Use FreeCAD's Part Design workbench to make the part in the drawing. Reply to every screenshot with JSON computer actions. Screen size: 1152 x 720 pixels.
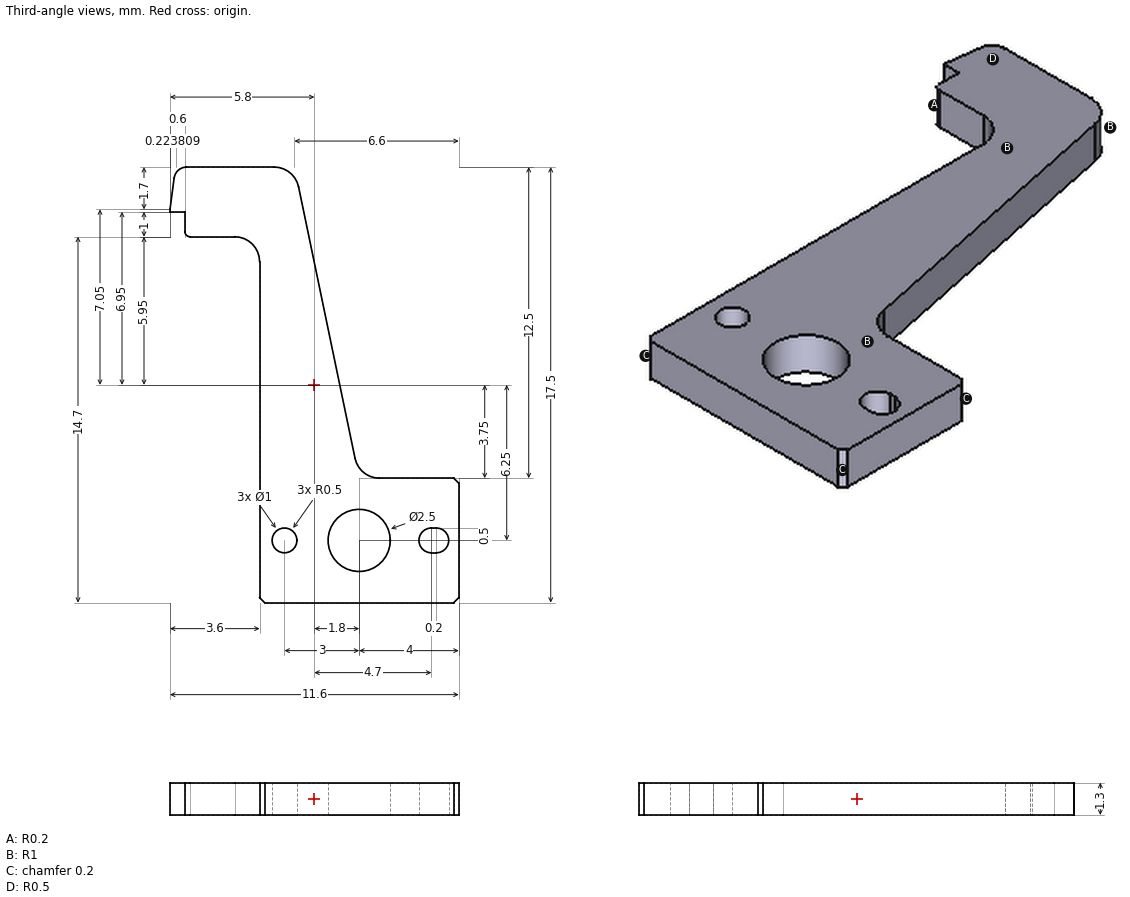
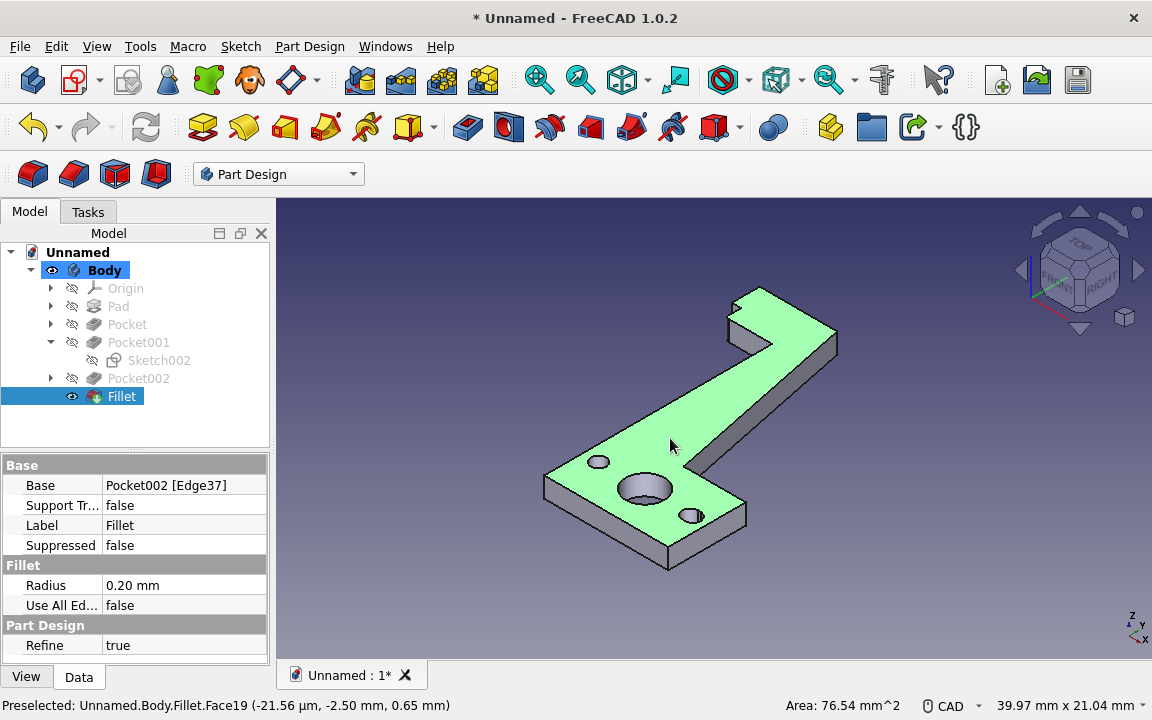
{"action": "left_click", "coordinate": [74, 80]}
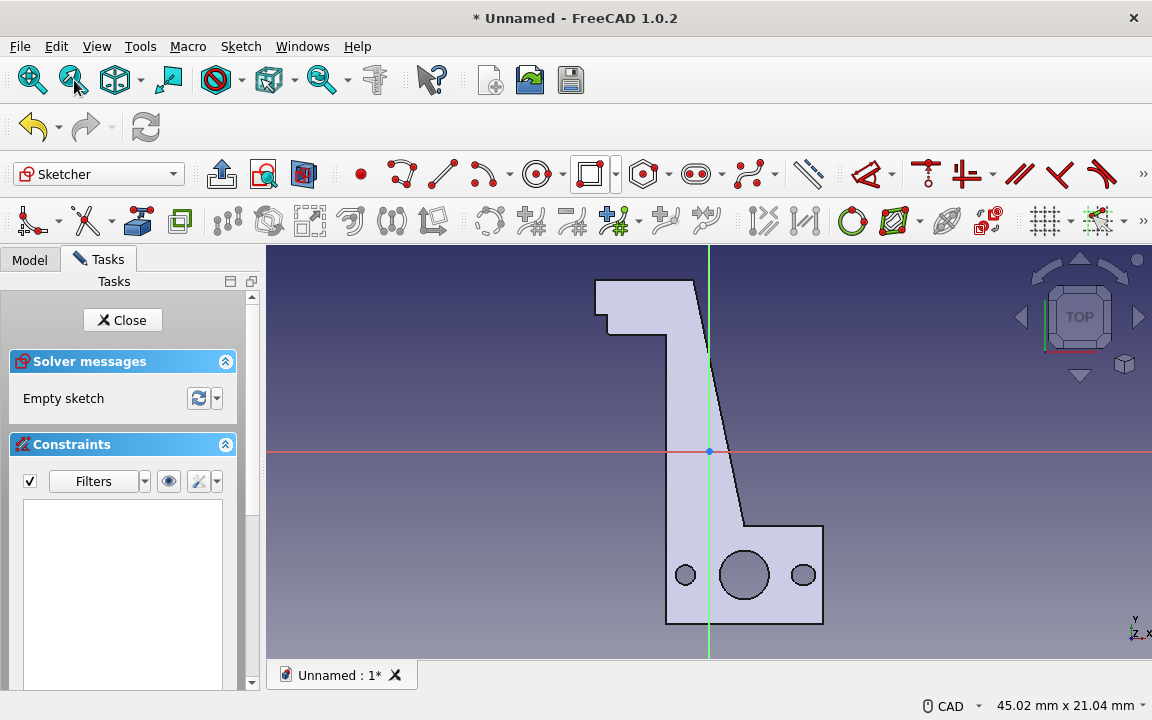
{"action": "scroll", "coordinate": [590, 273], "scroll_direction": "up", "scroll_amount": 10}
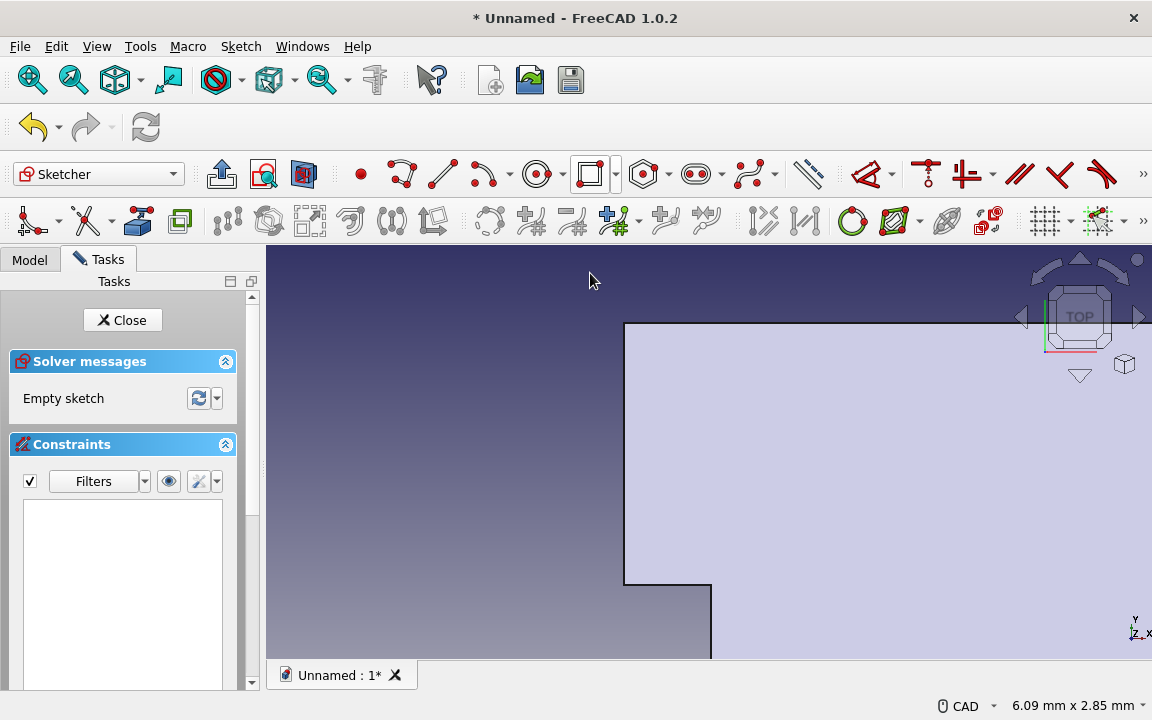
{"action": "key", "text": "g m"}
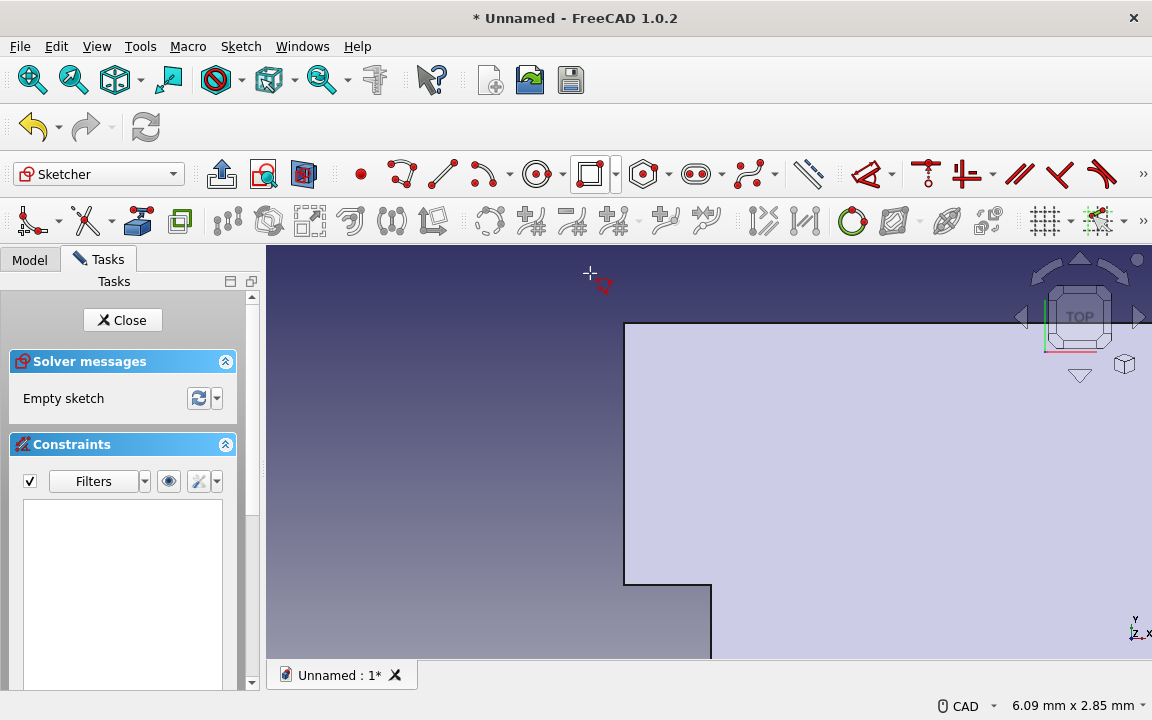
{"action": "left_click", "coordinate": [624, 570]}
{"action": "left_click", "coordinate": [656, 323]}
{"action": "left_click", "coordinate": [624, 323]}
{"action": "left_click", "coordinate": [624, 571]}
{"action": "key", "text": "Escape"}
{"action": "key", "text": "Escape"}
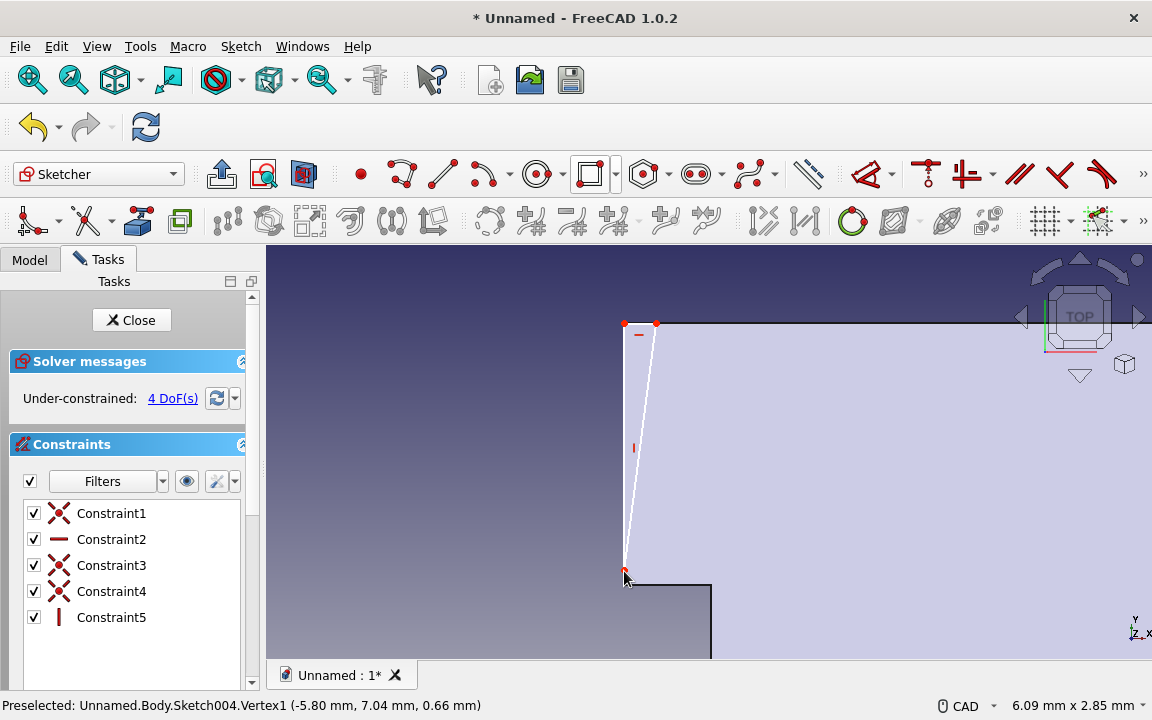
{"action": "key", "text": "d"}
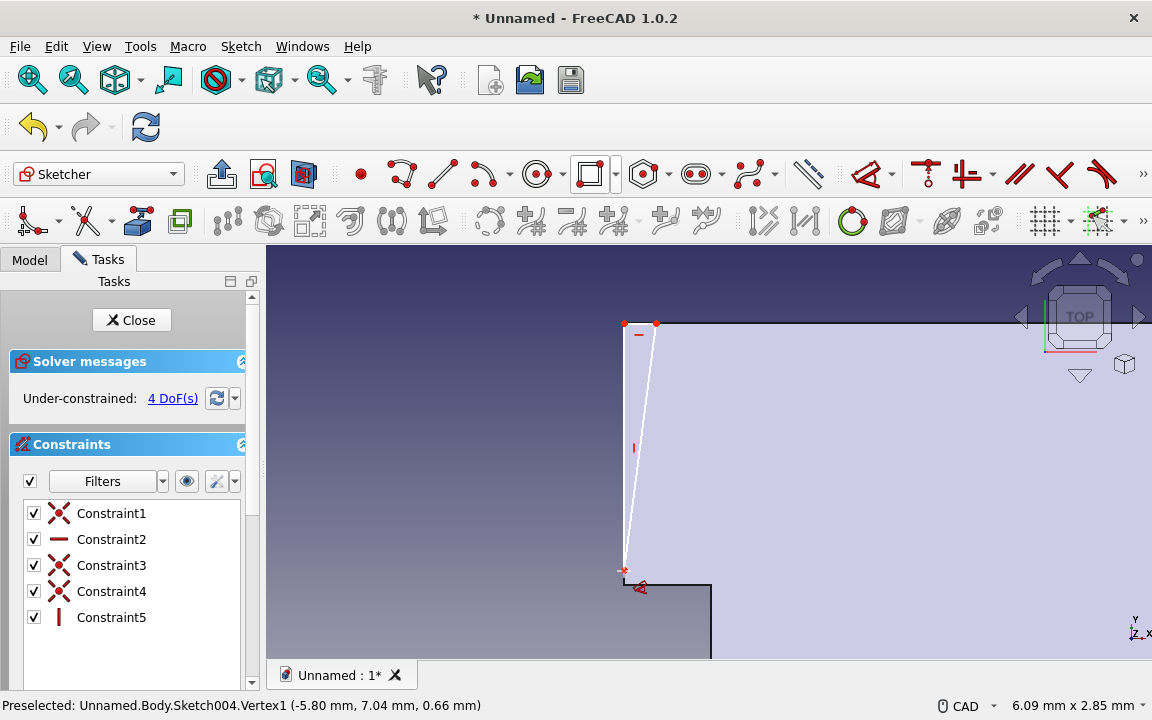
{"action": "left_click", "coordinate": [624, 398]}
{"action": "left_click", "coordinate": [590, 447]}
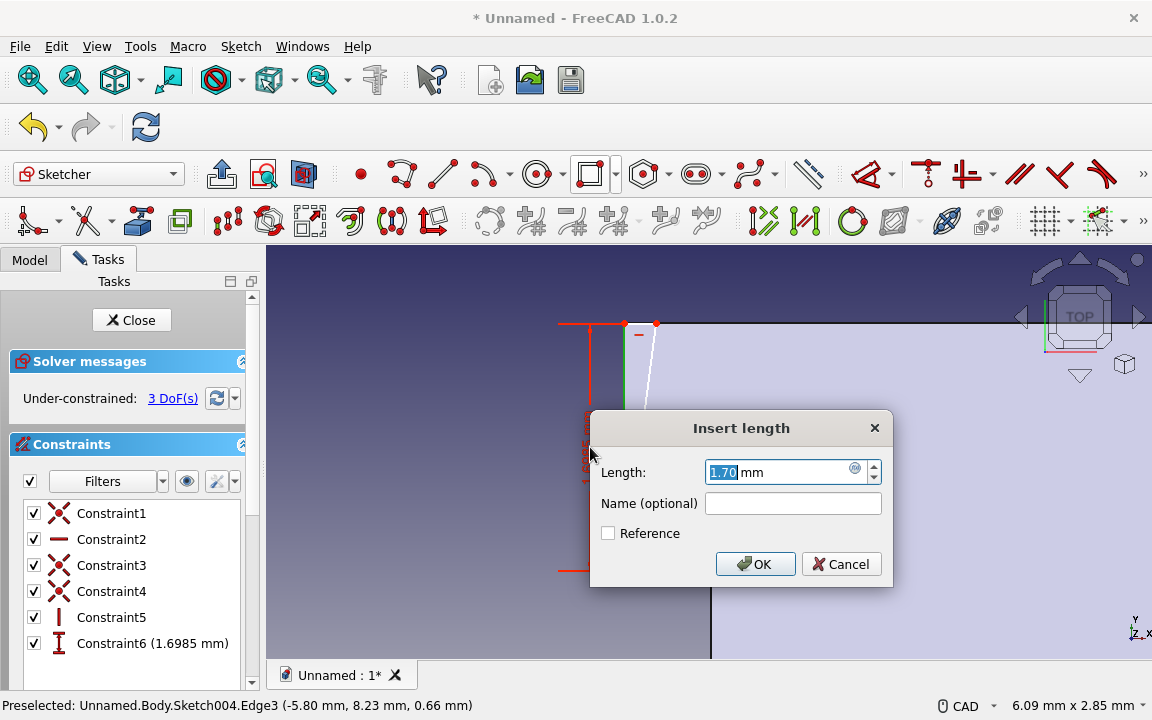
{"action": "type", "text": "1.7"}
{"action": "key", "text": "Return"}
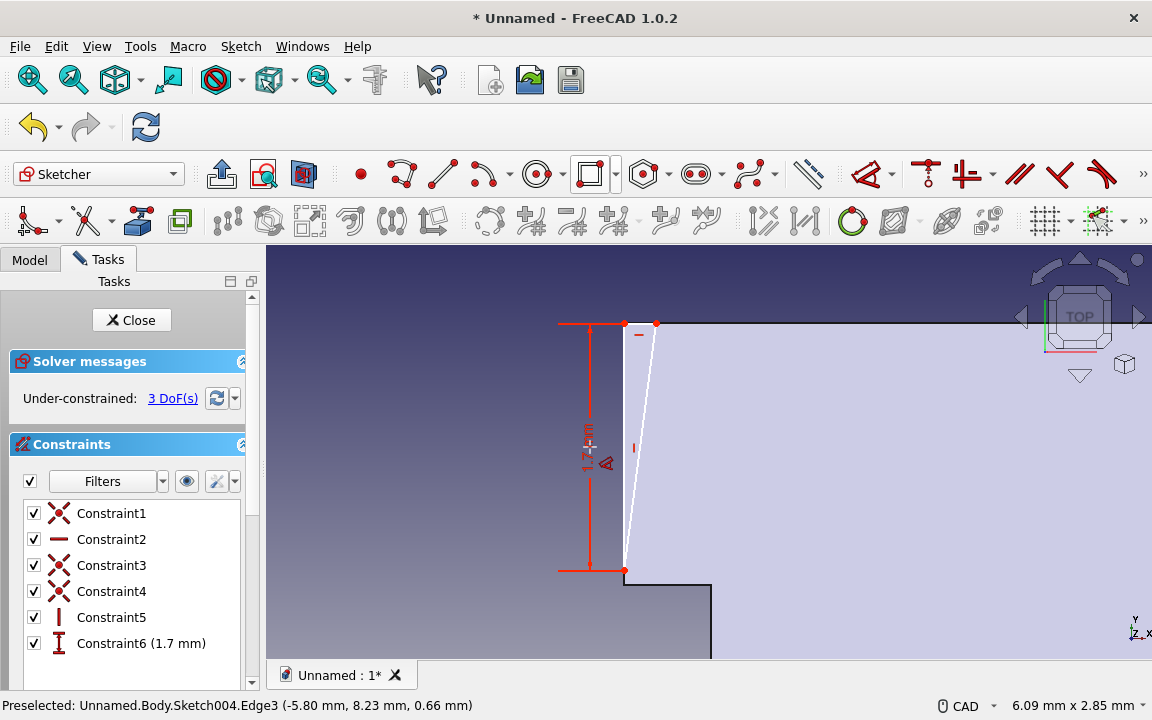
{"action": "left_click", "coordinate": [624, 571]}
{"action": "left_click", "coordinate": [805, 537]}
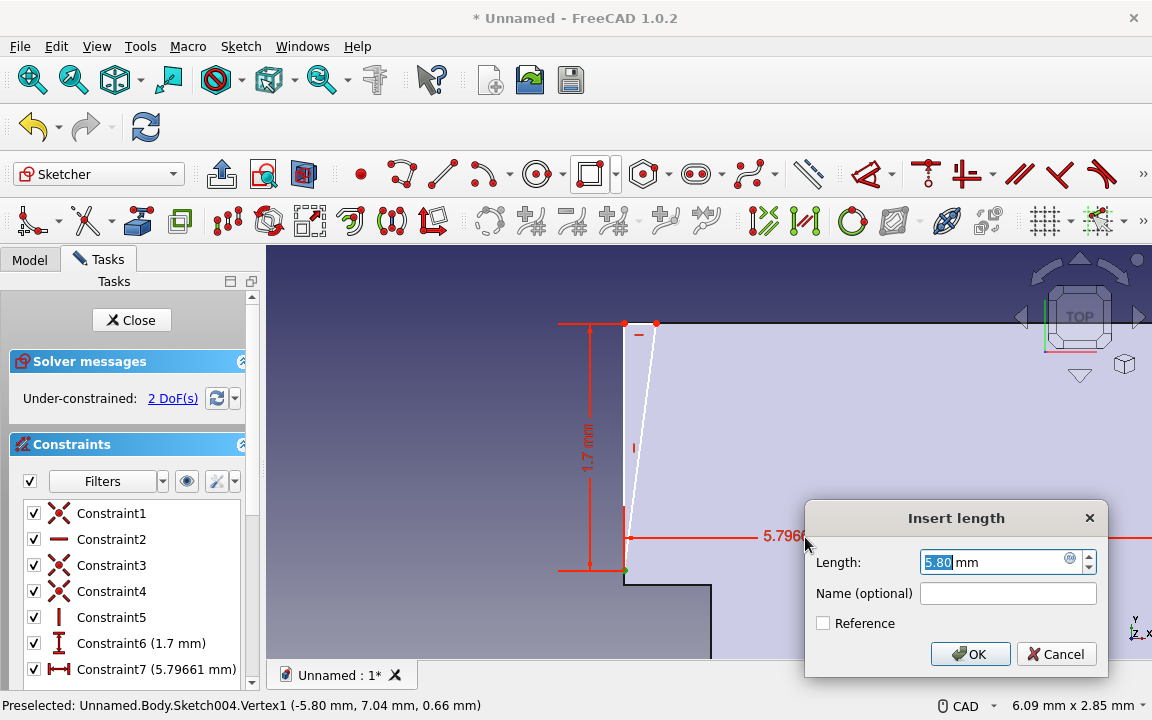
{"action": "type", "text": "5.8"}
{"action": "key", "text": "Return"}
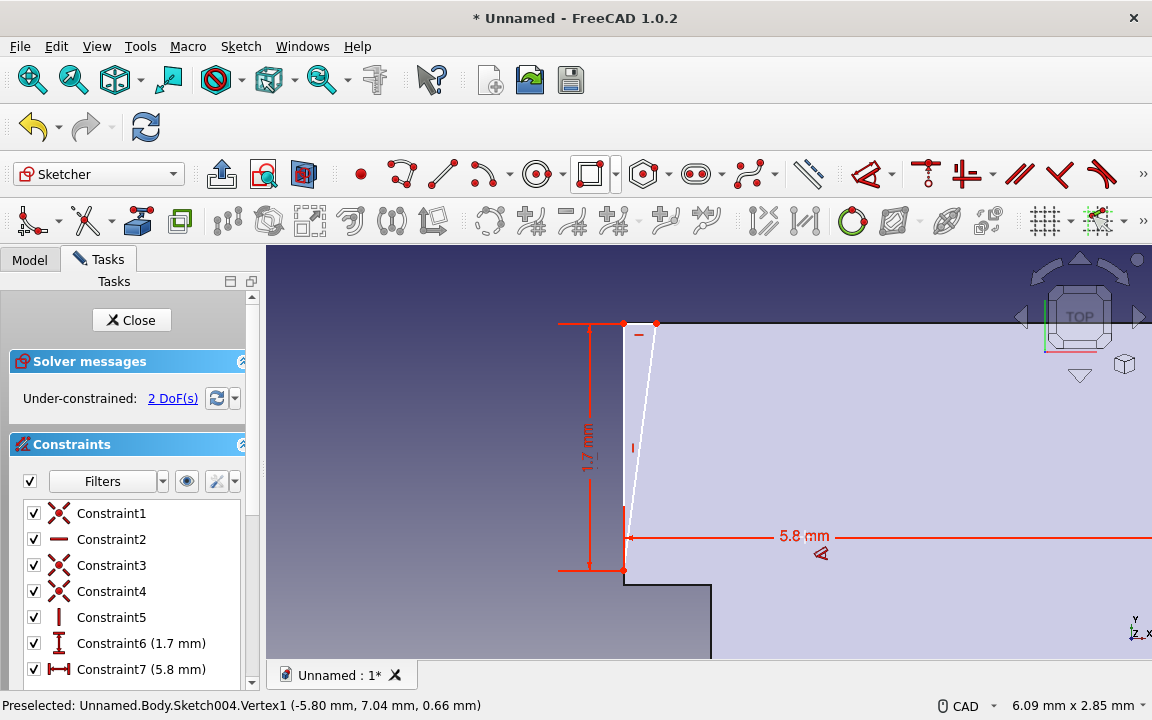
{"action": "left_click", "coordinate": [624, 571]}
{"action": "left_click", "coordinate": [590, 601]}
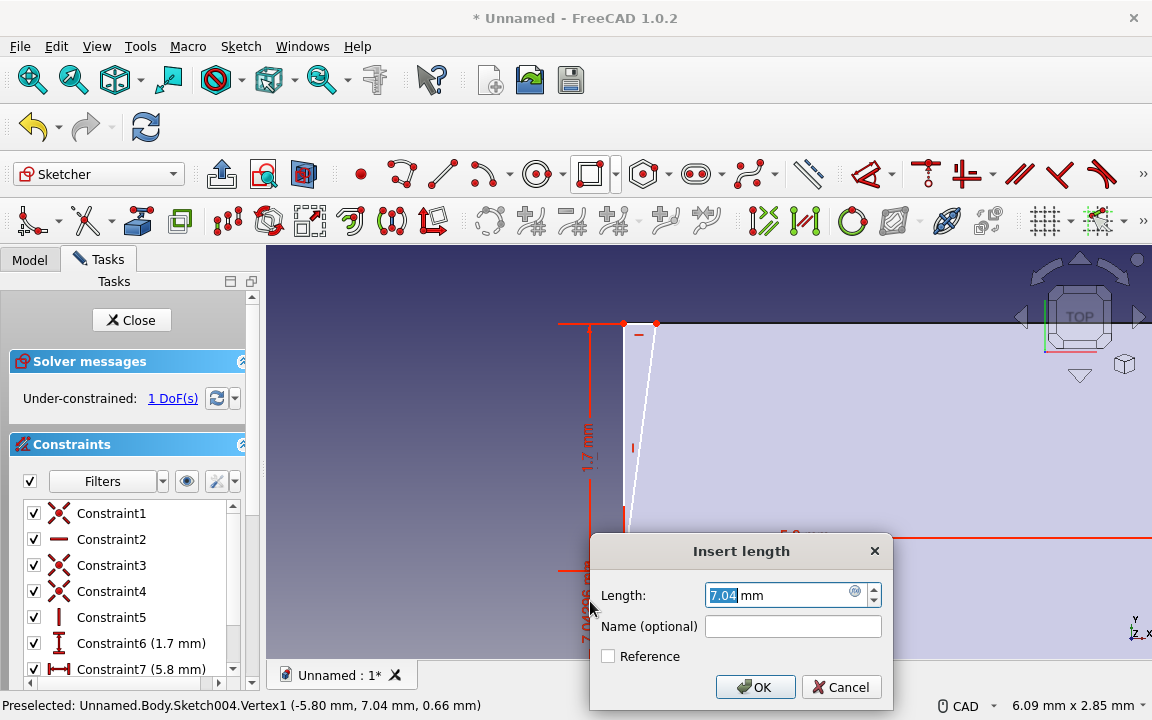
{"action": "type", "text": "7.05"}
{"action": "key", "text": "Return"}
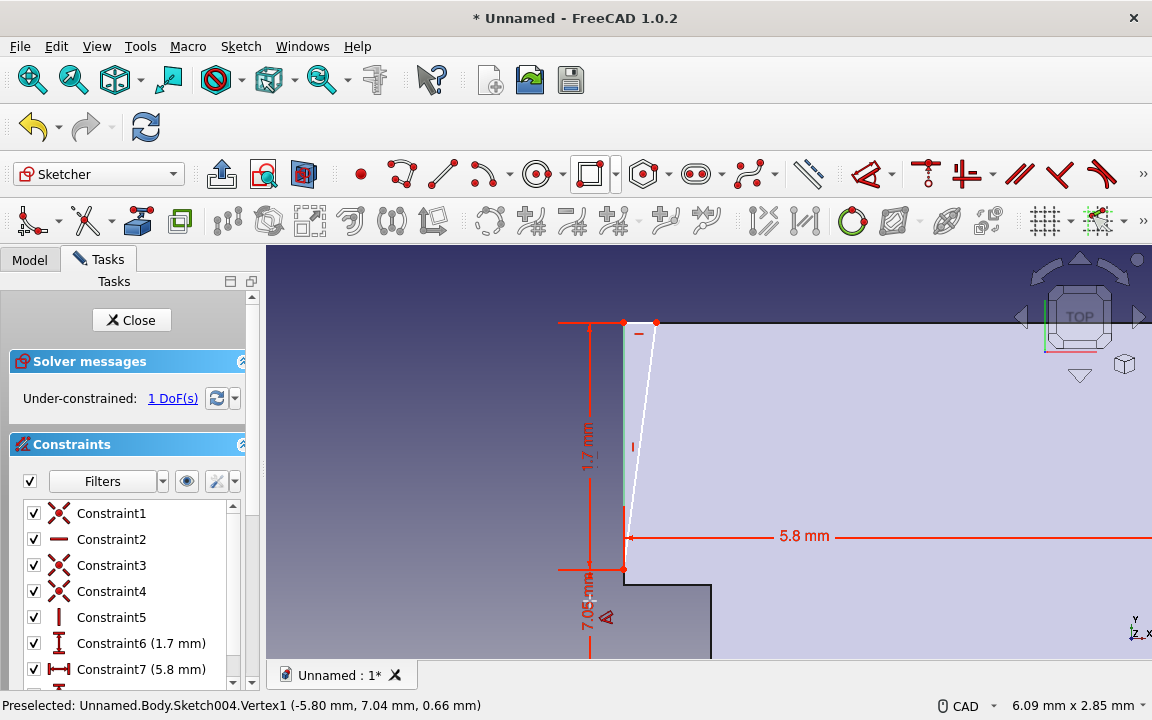
{"action": "scroll", "coordinate": [646, 323], "scroll_direction": "up", "scroll_amount": 2}